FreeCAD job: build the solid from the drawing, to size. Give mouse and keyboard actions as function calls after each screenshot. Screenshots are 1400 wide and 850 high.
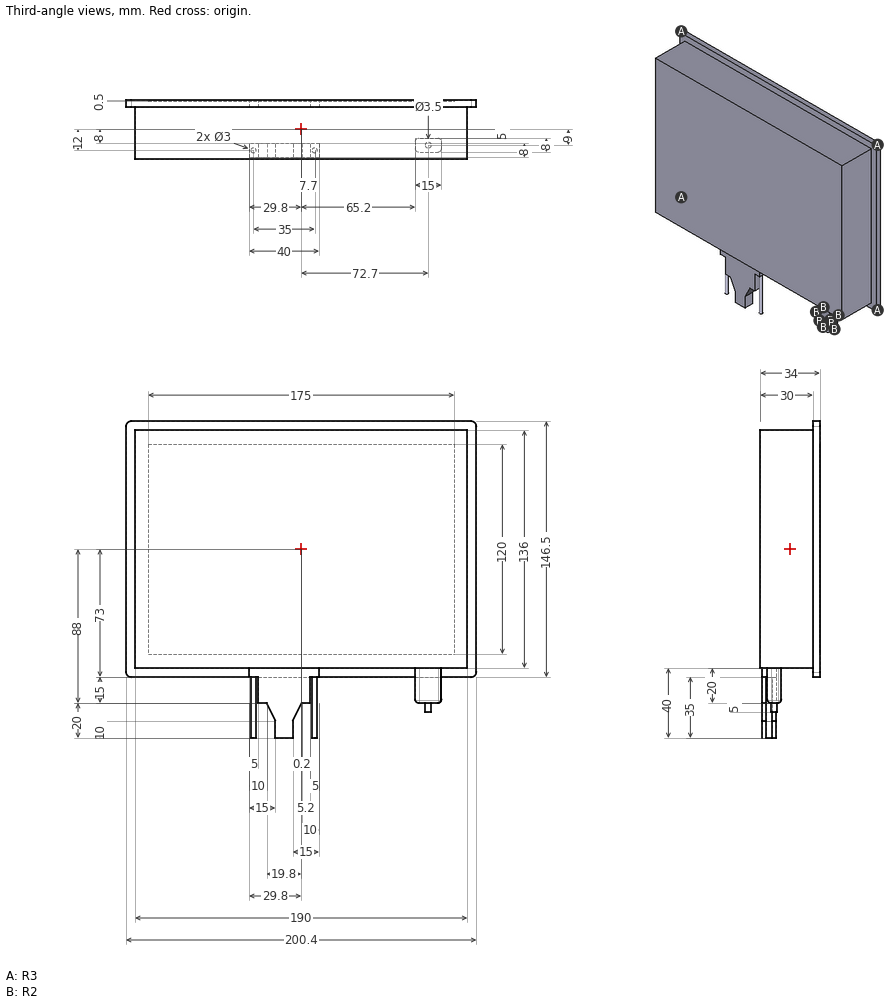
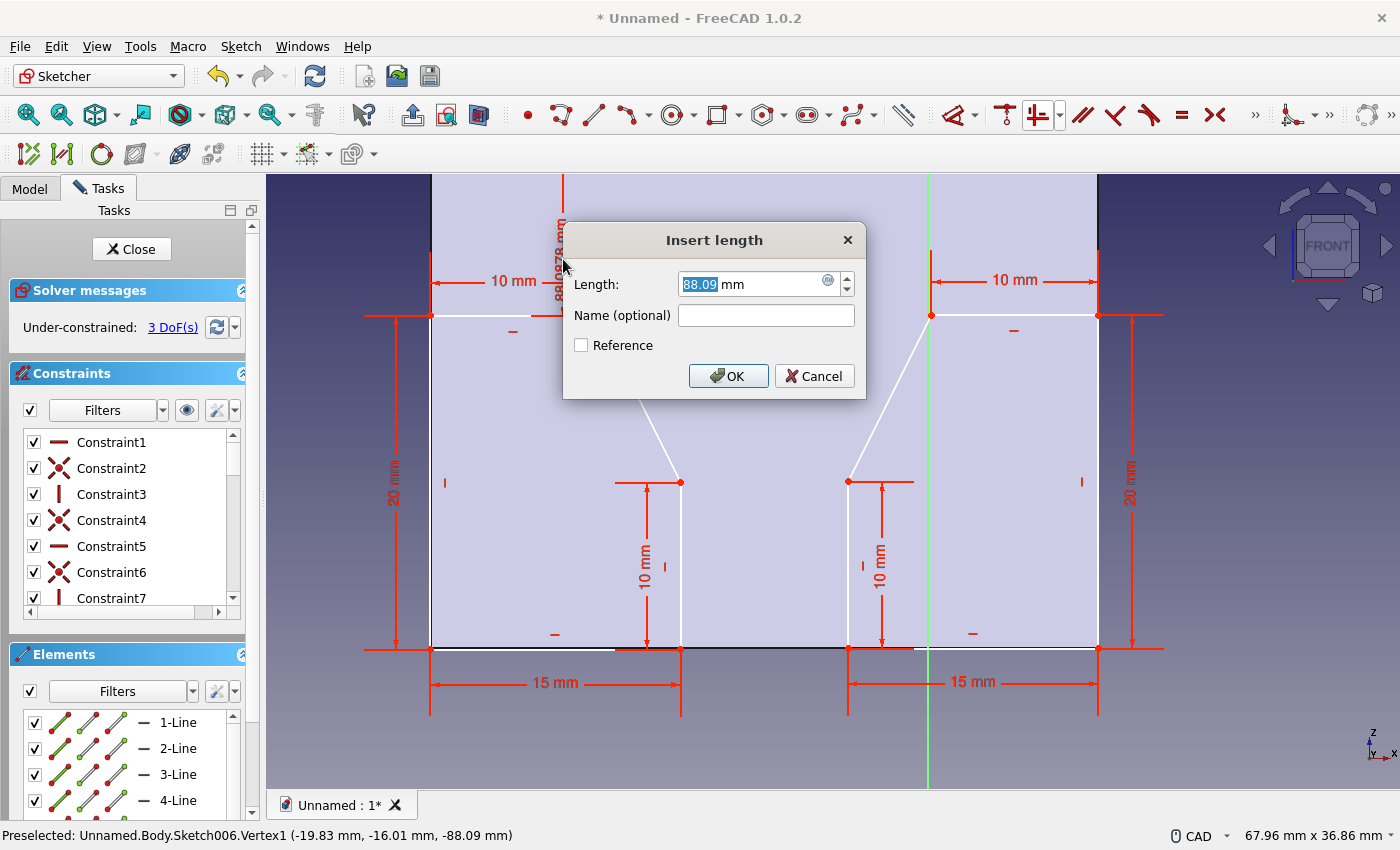
text(88)
key(Return)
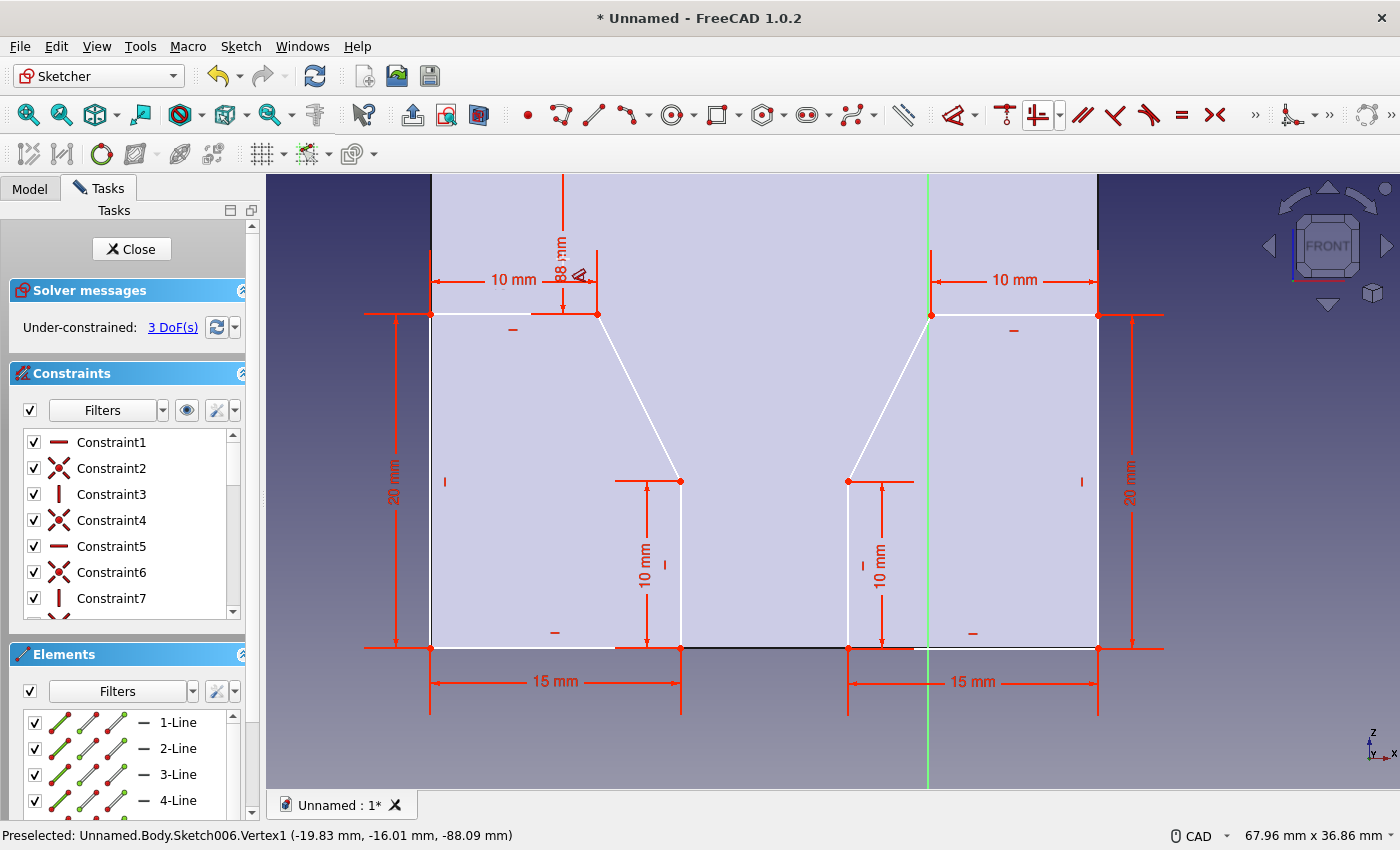
click(931, 315)
click(965, 259)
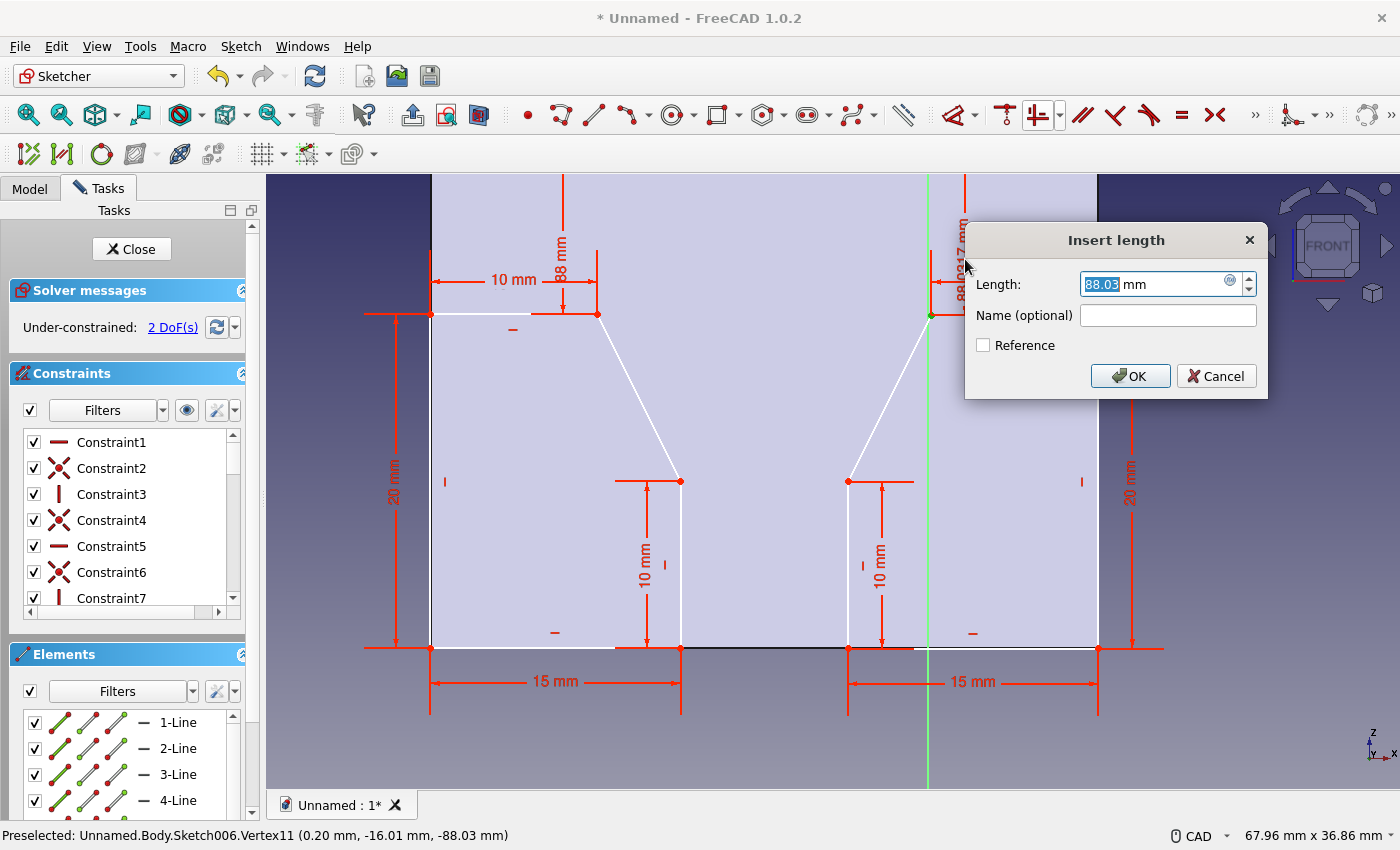
text(88)
key(Return)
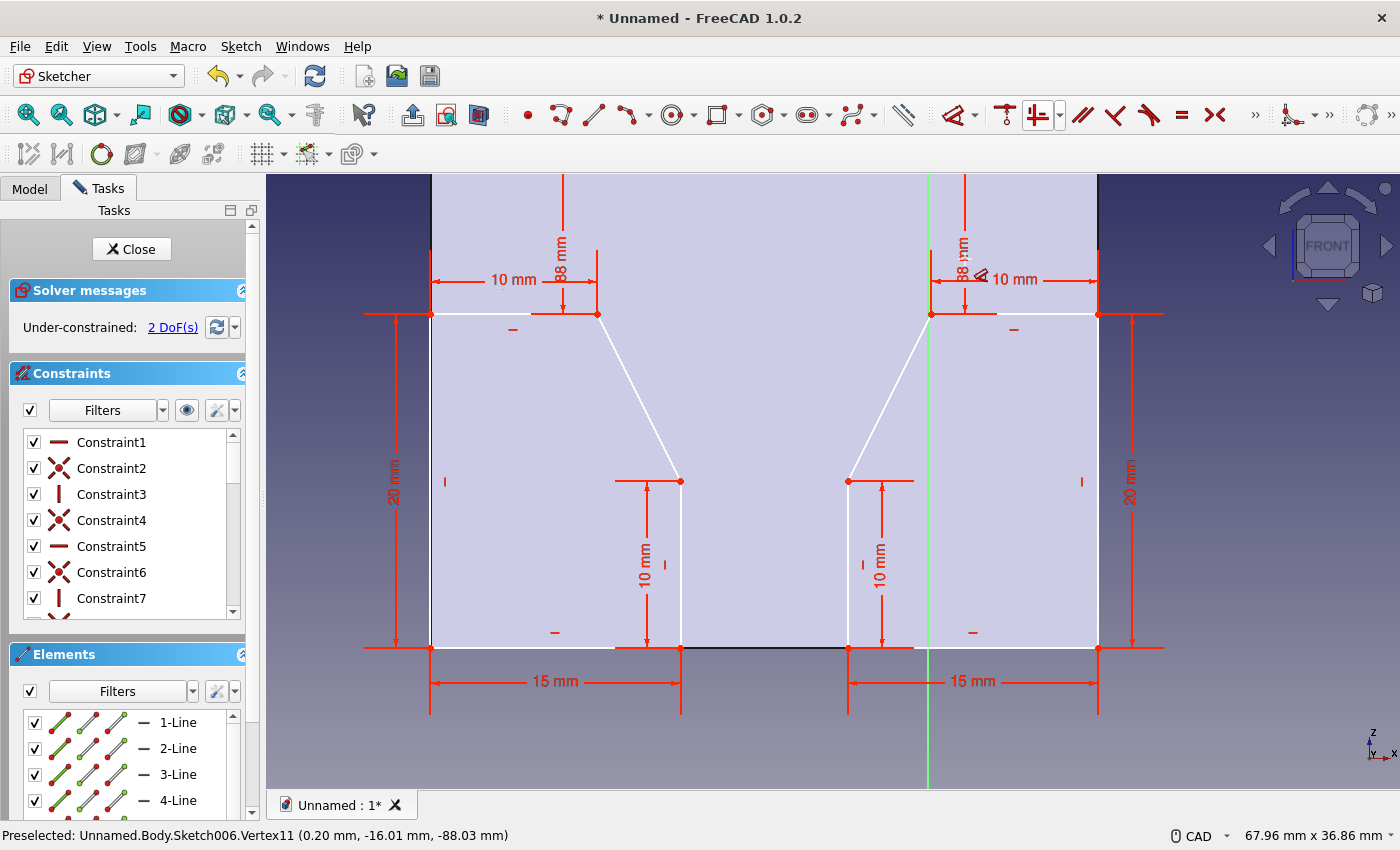
scroll(931, 314, up, 13)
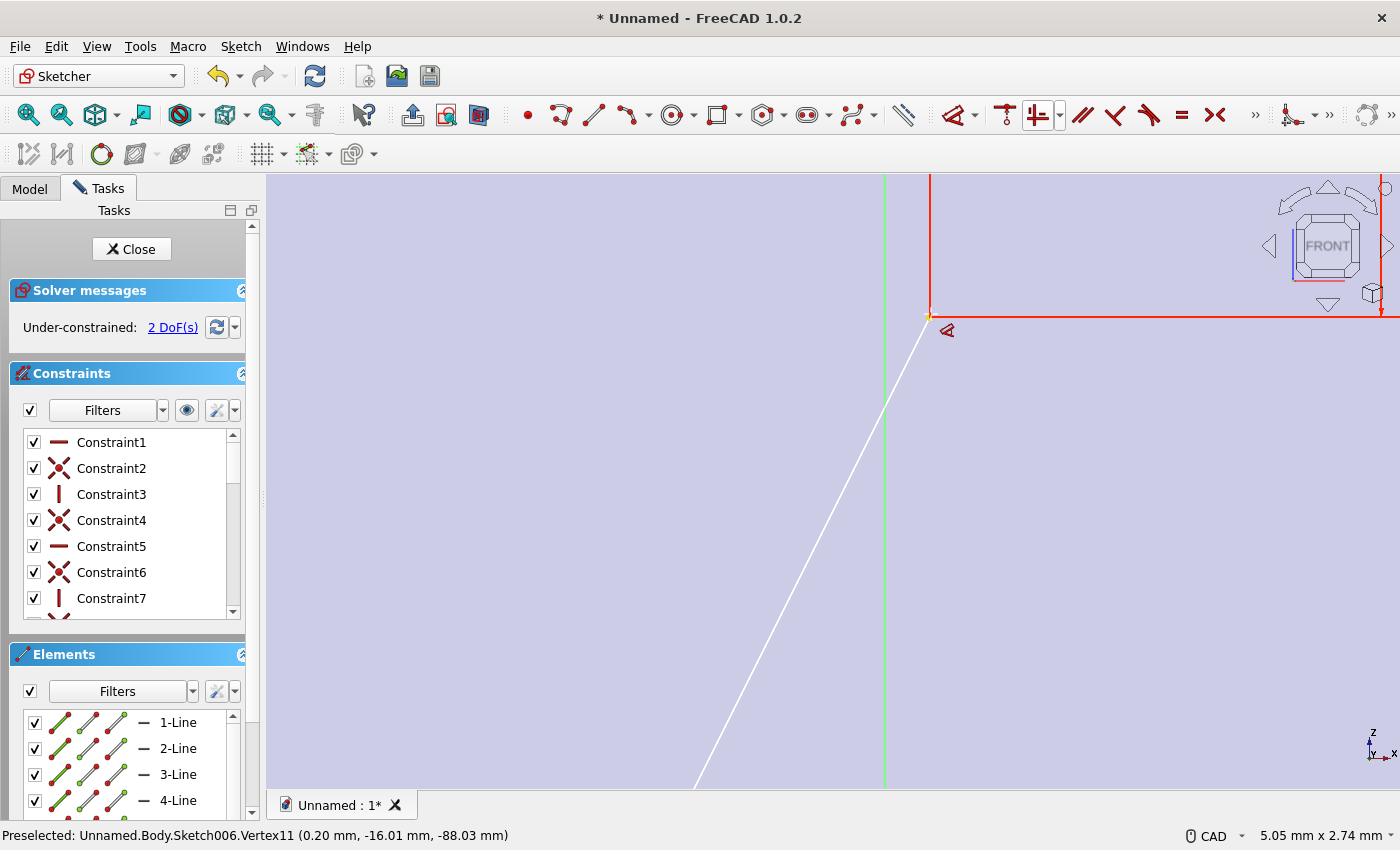
click(930, 317)
click(918, 375)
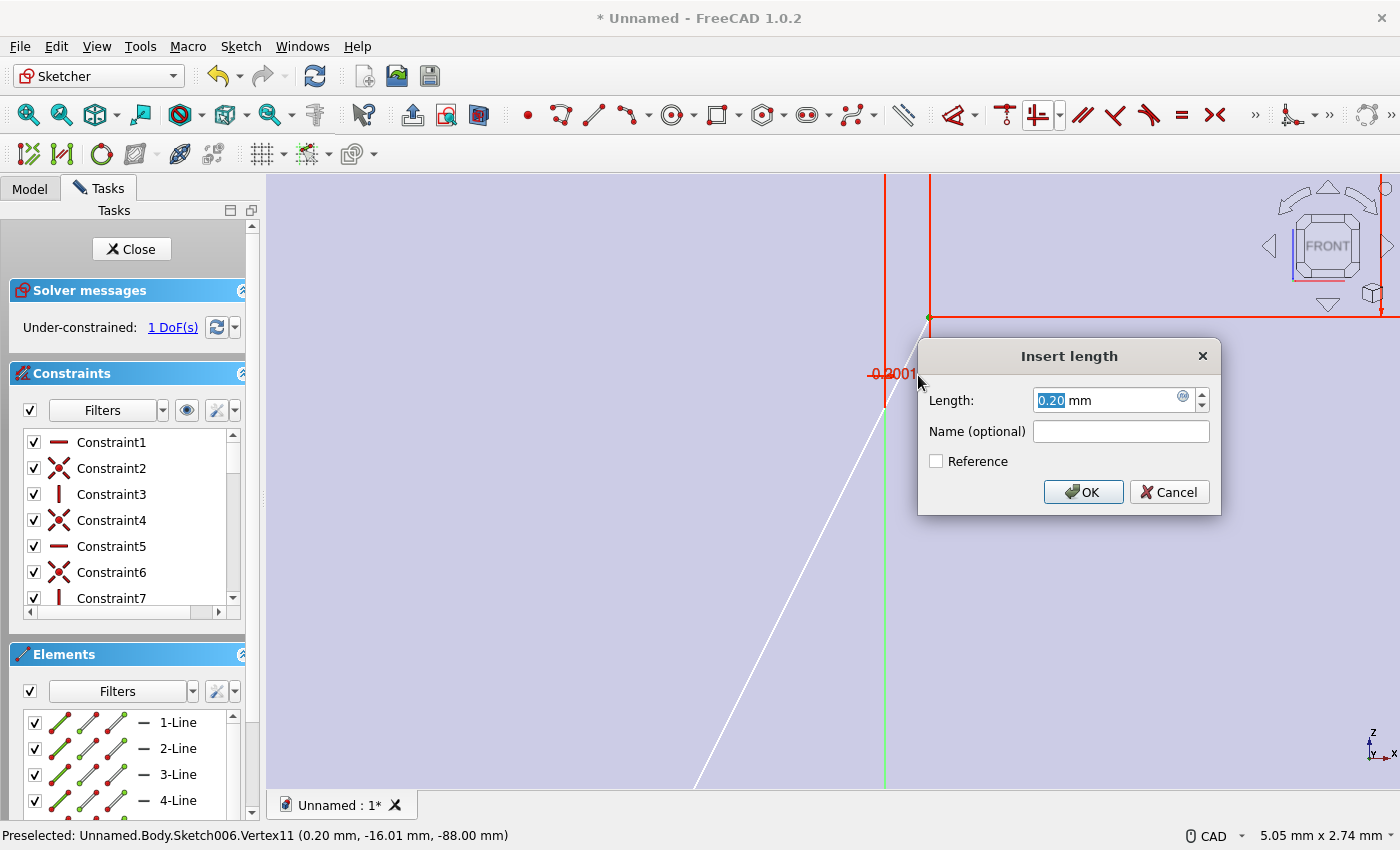
text(0.2)
key(Return)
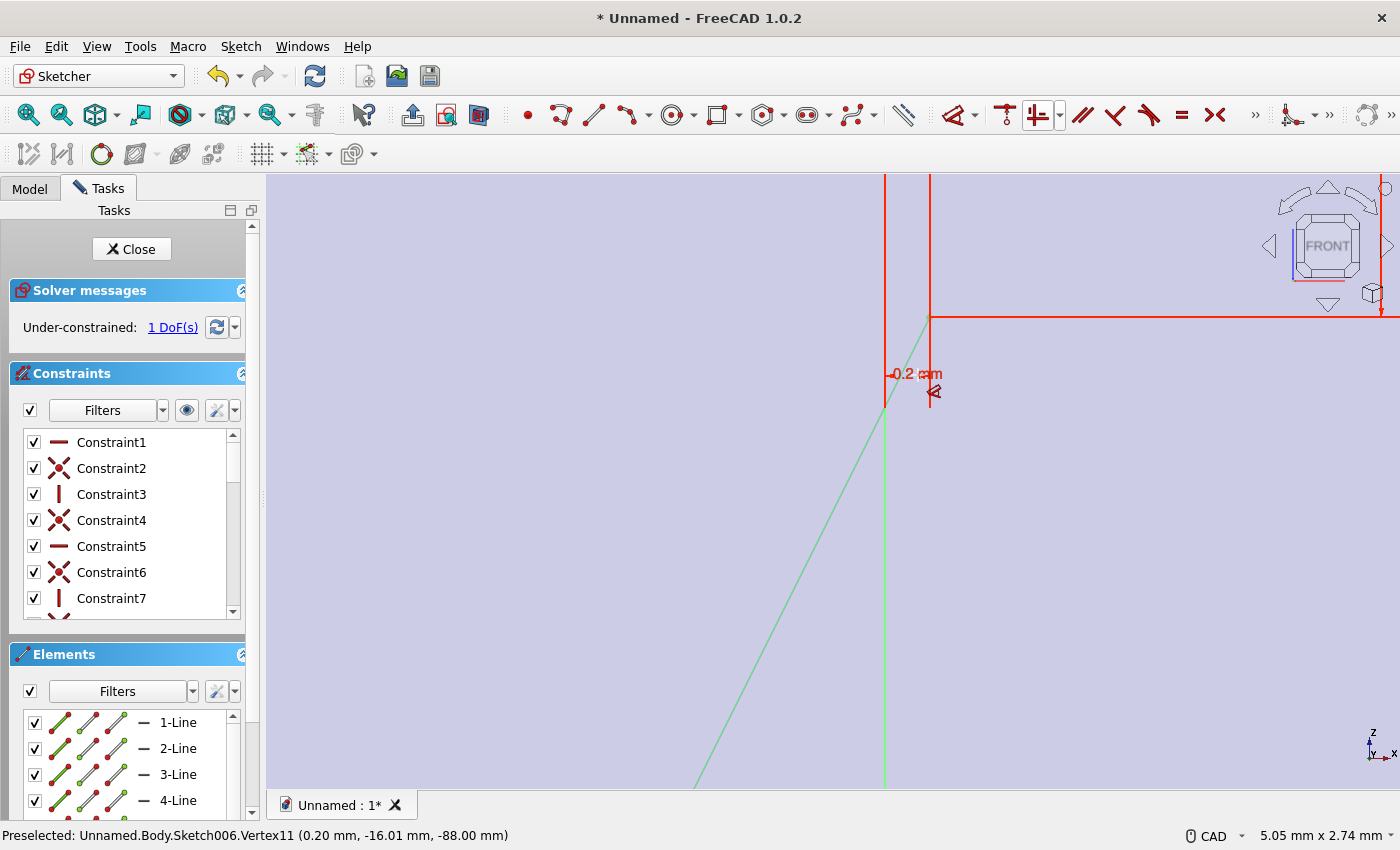
scroll(931, 314, down, 13)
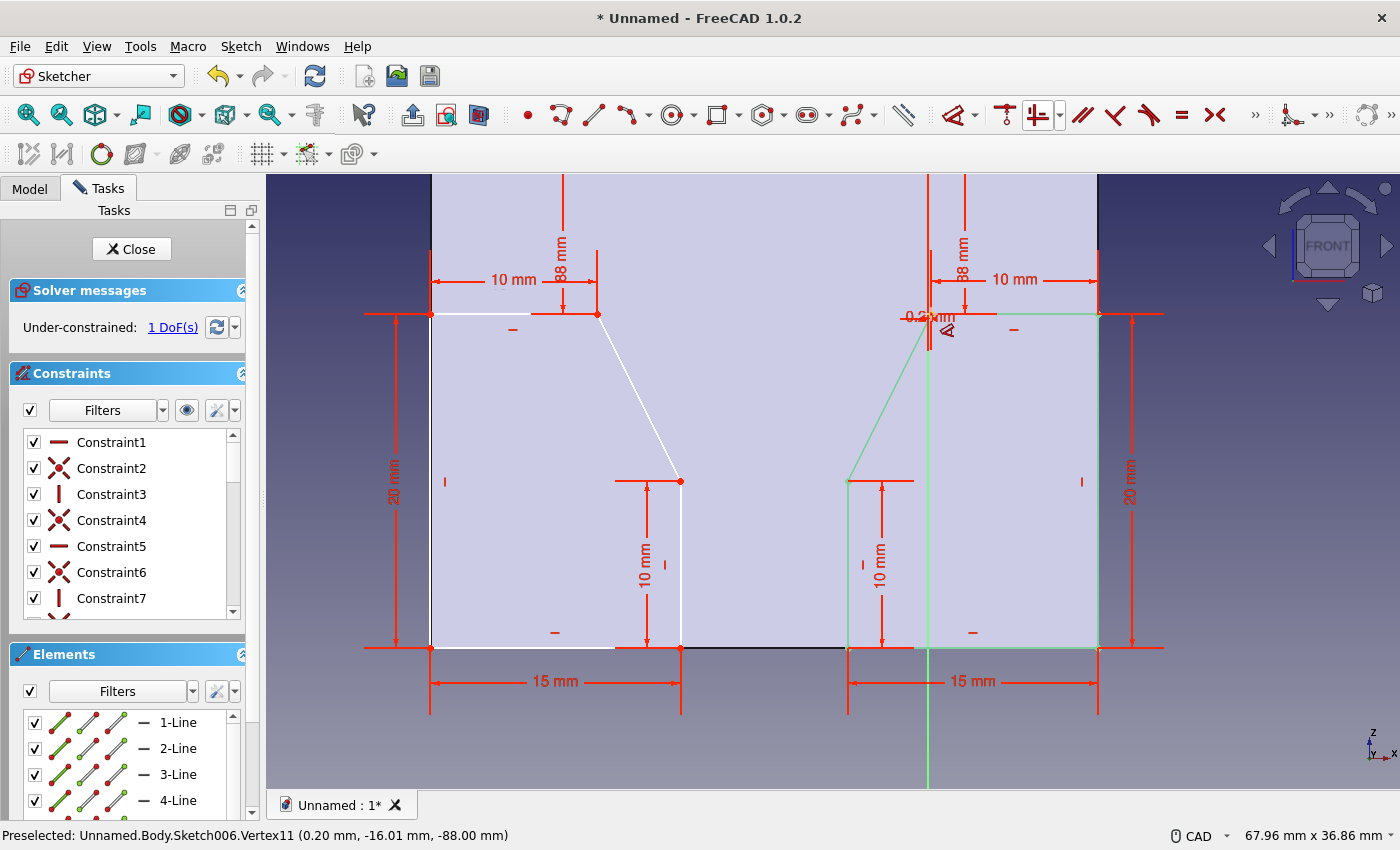
click(597, 314)
click(763, 348)